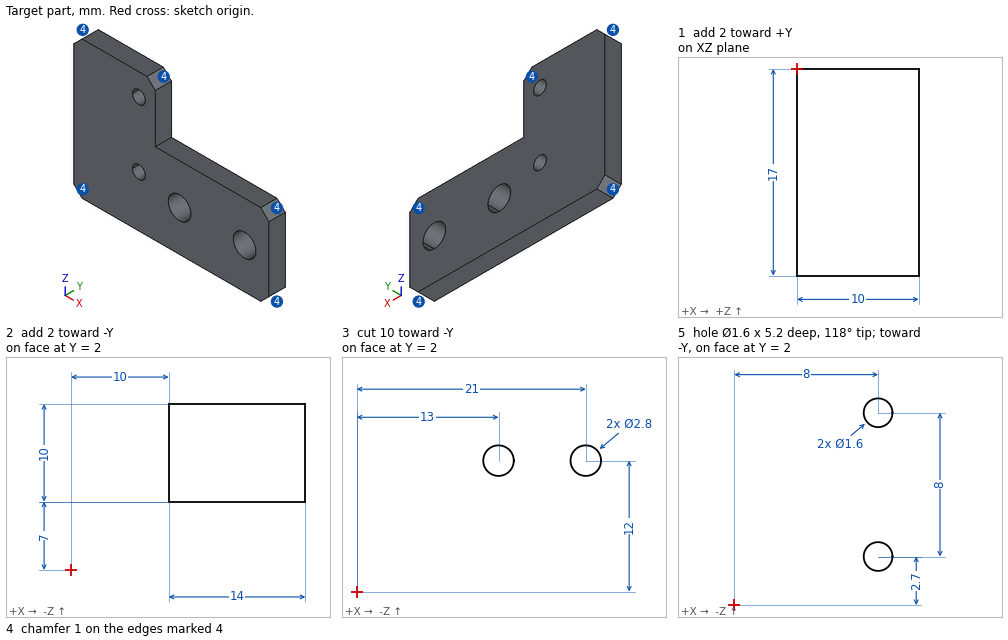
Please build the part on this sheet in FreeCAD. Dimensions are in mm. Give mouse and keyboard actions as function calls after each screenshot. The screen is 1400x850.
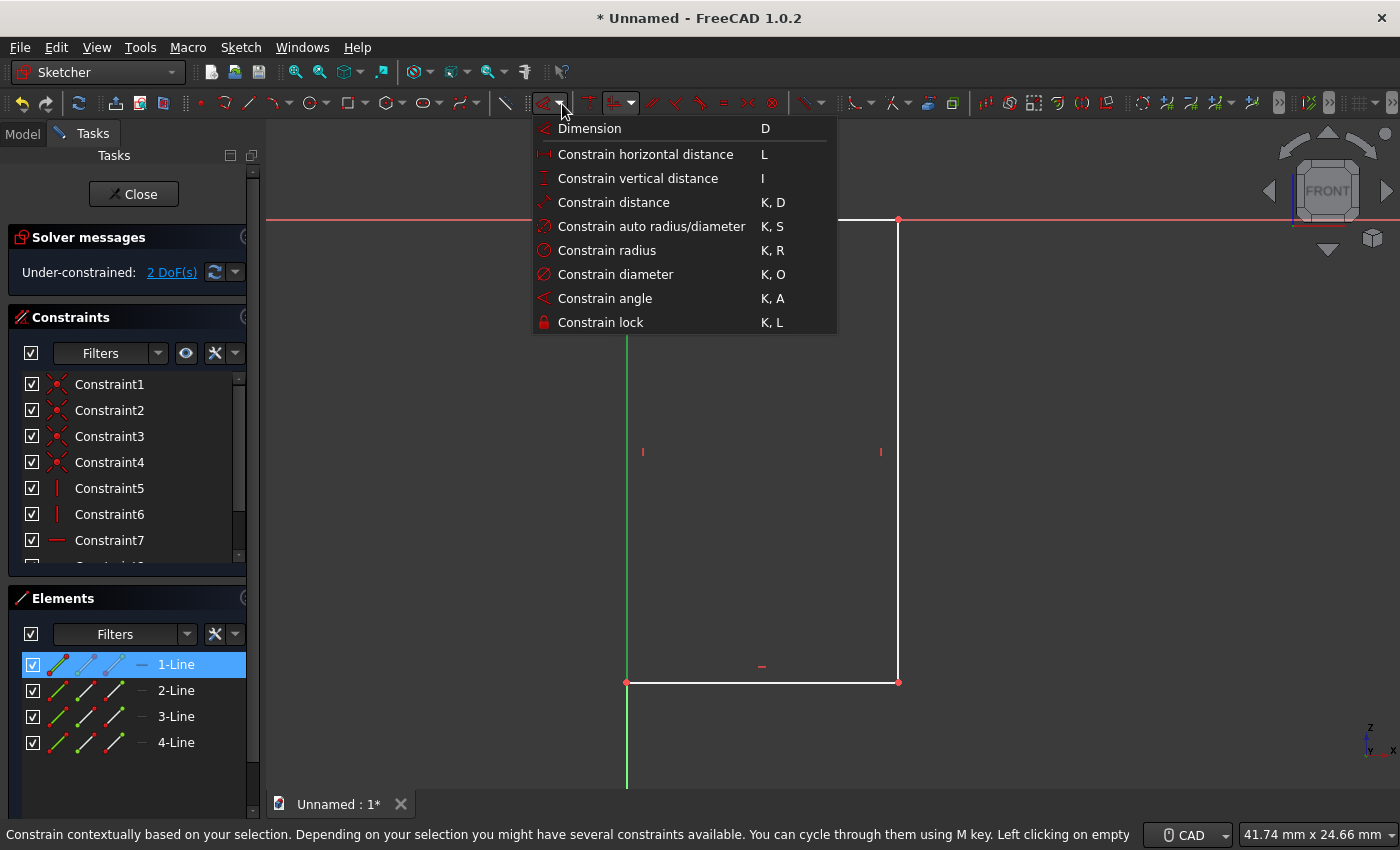
click(685, 178)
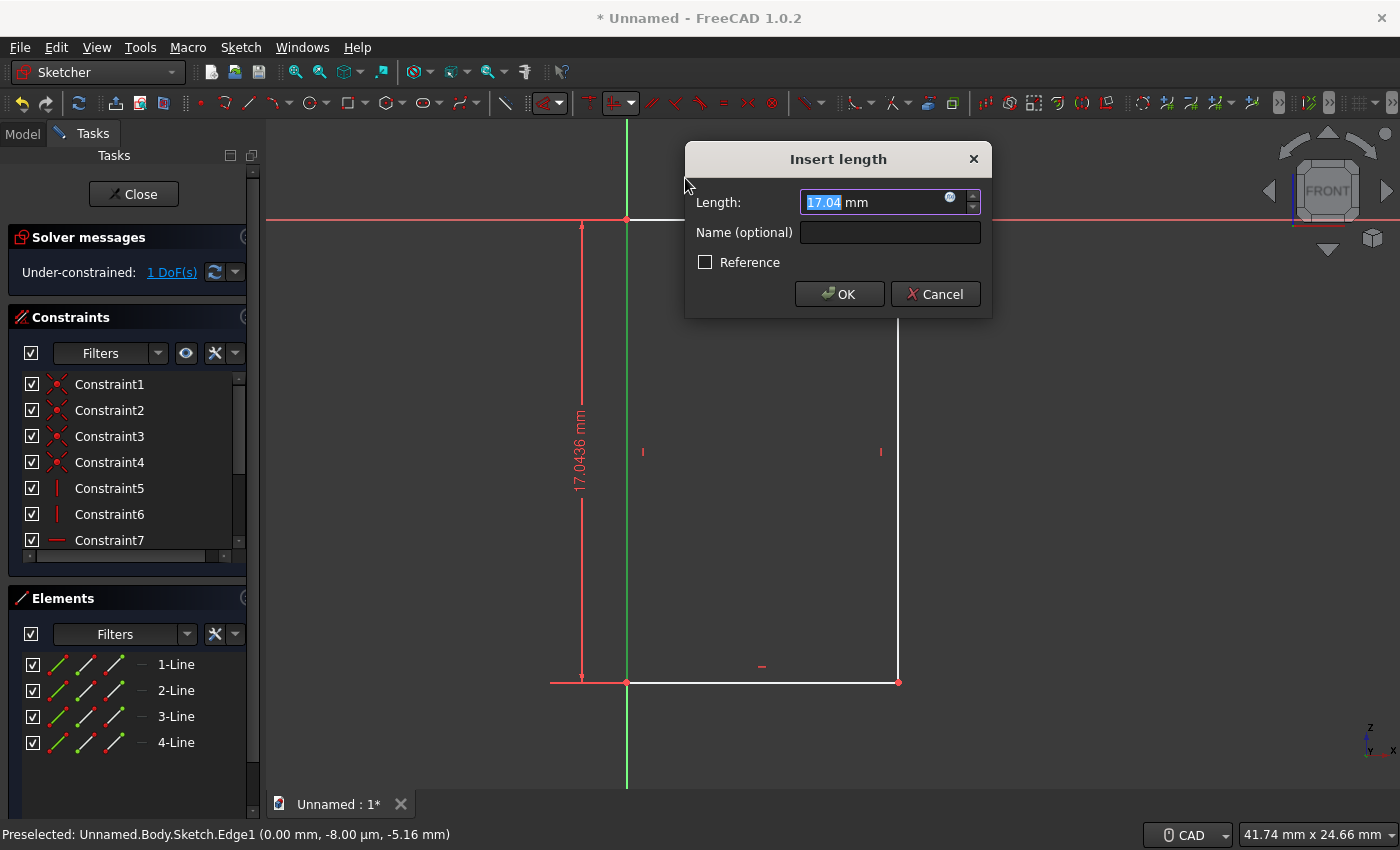
text(17)
key(Return)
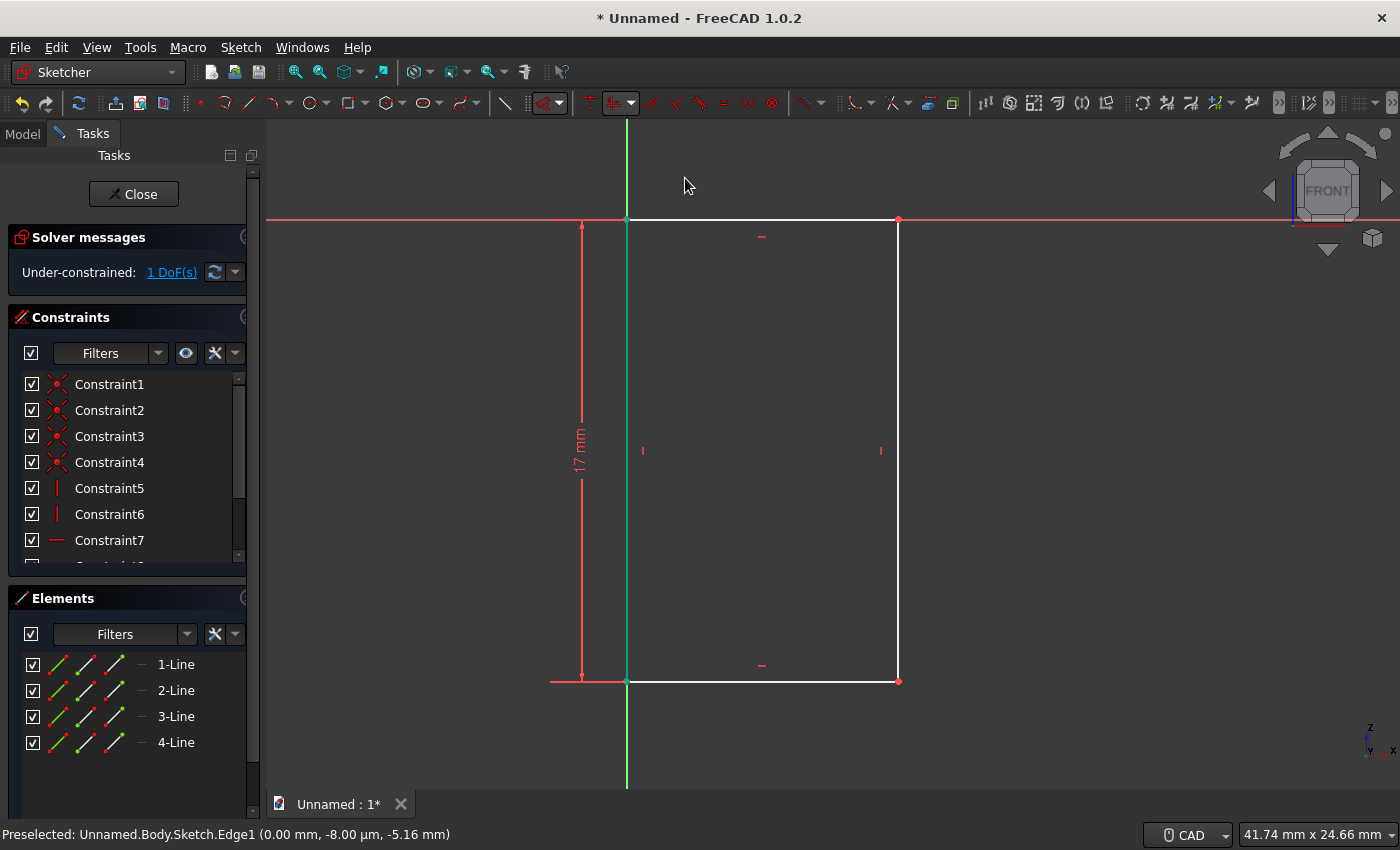
click(708, 682)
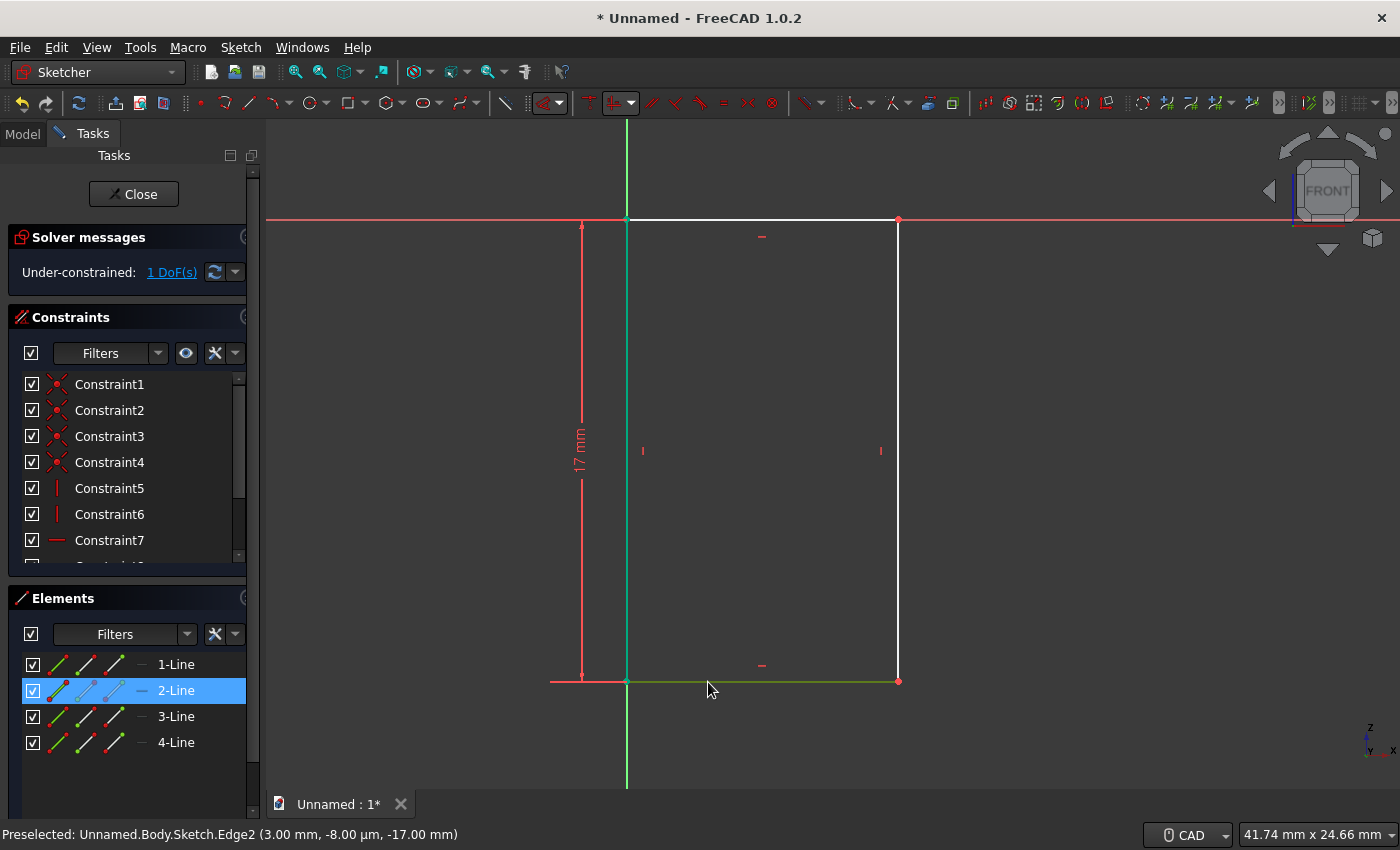
key(l)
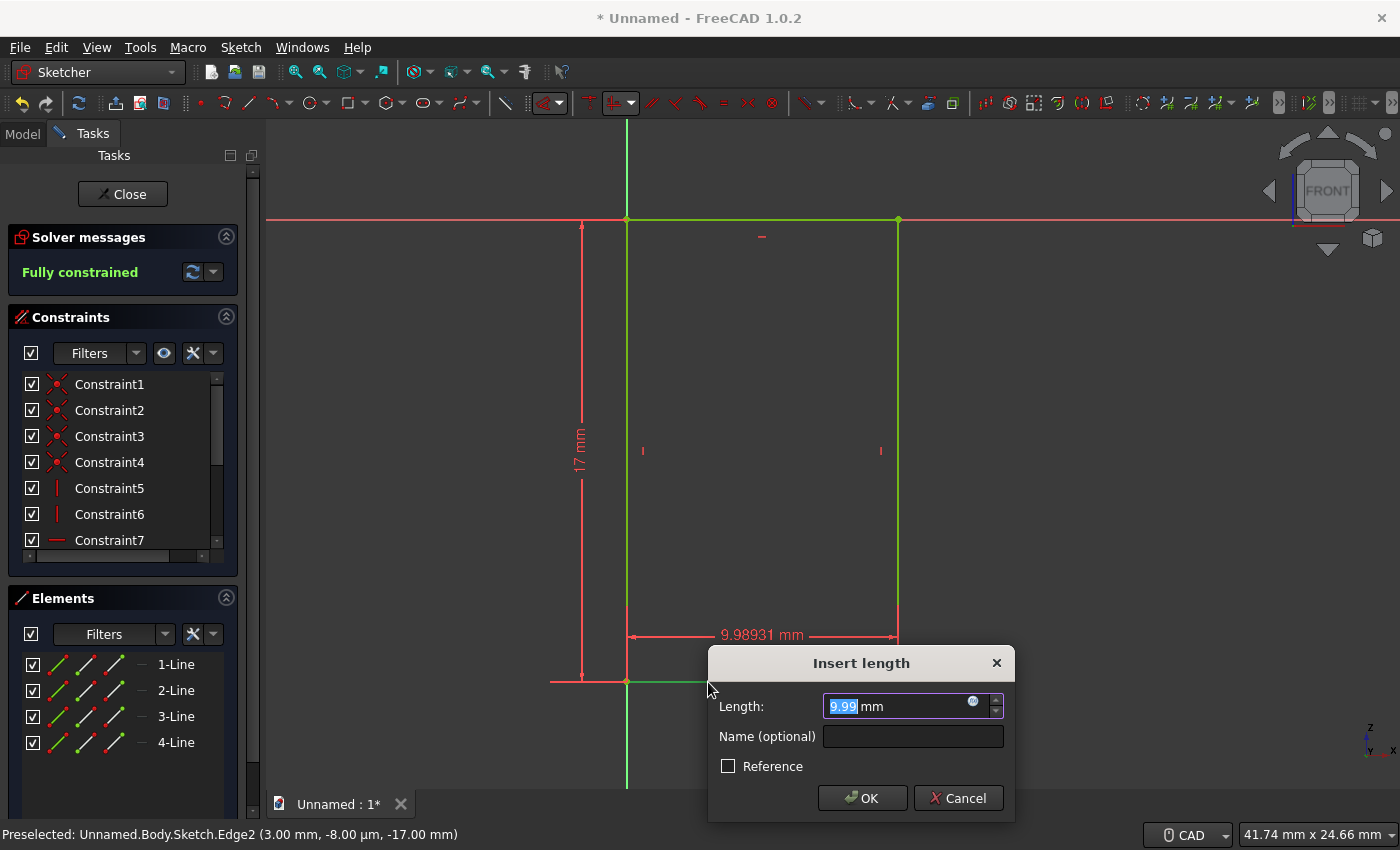
text(10)
key(Return)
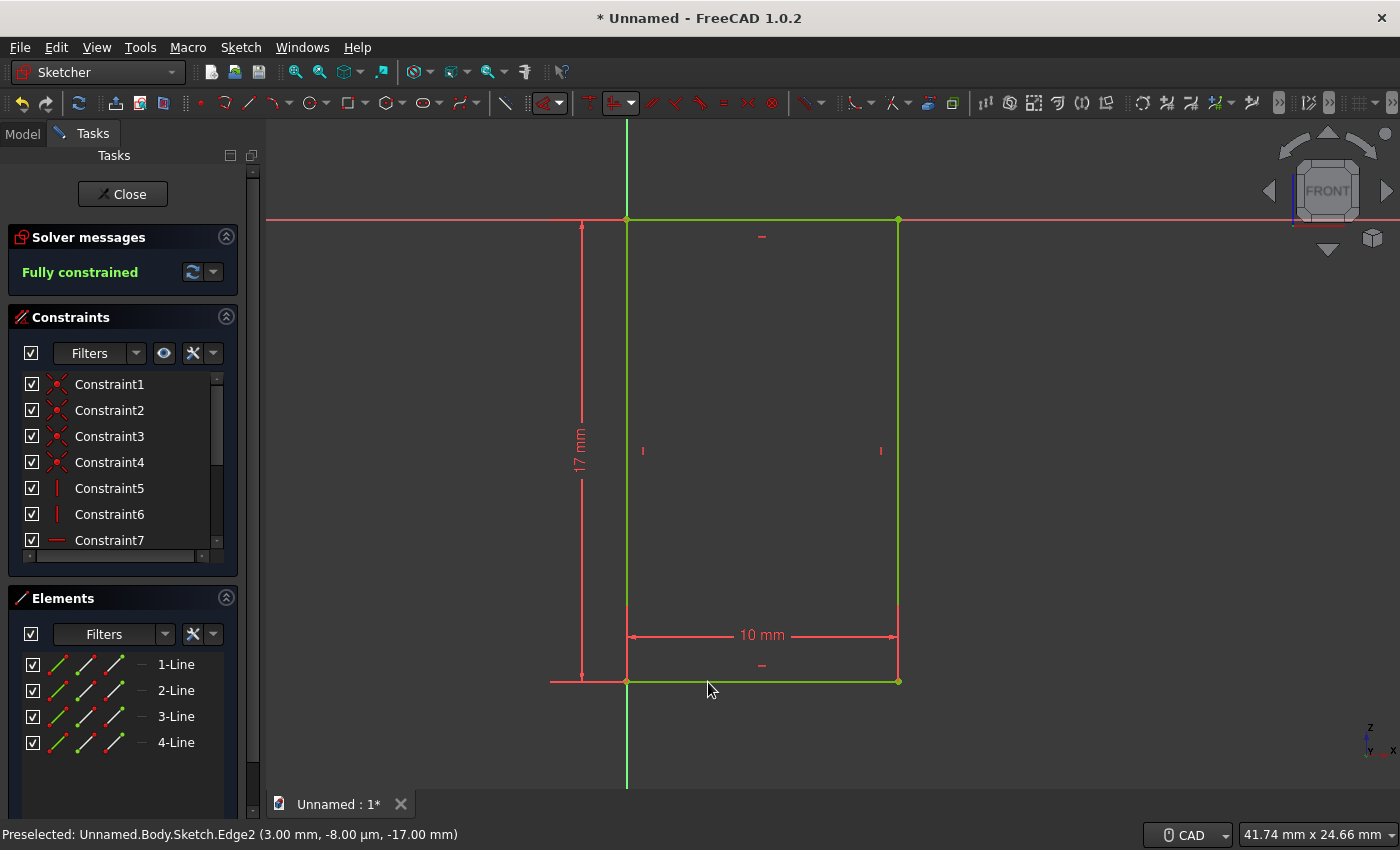
click(123, 194)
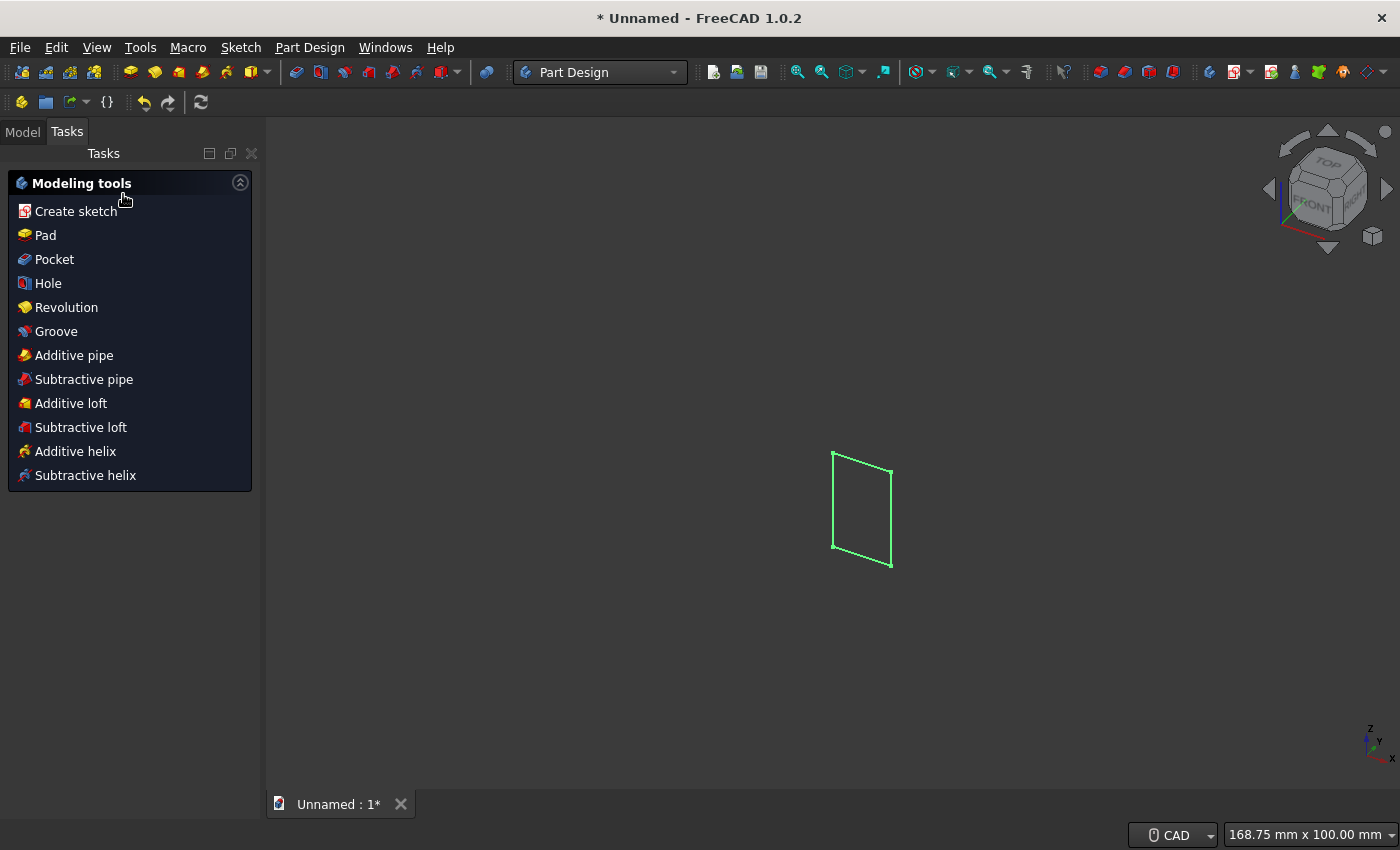
click(132, 72)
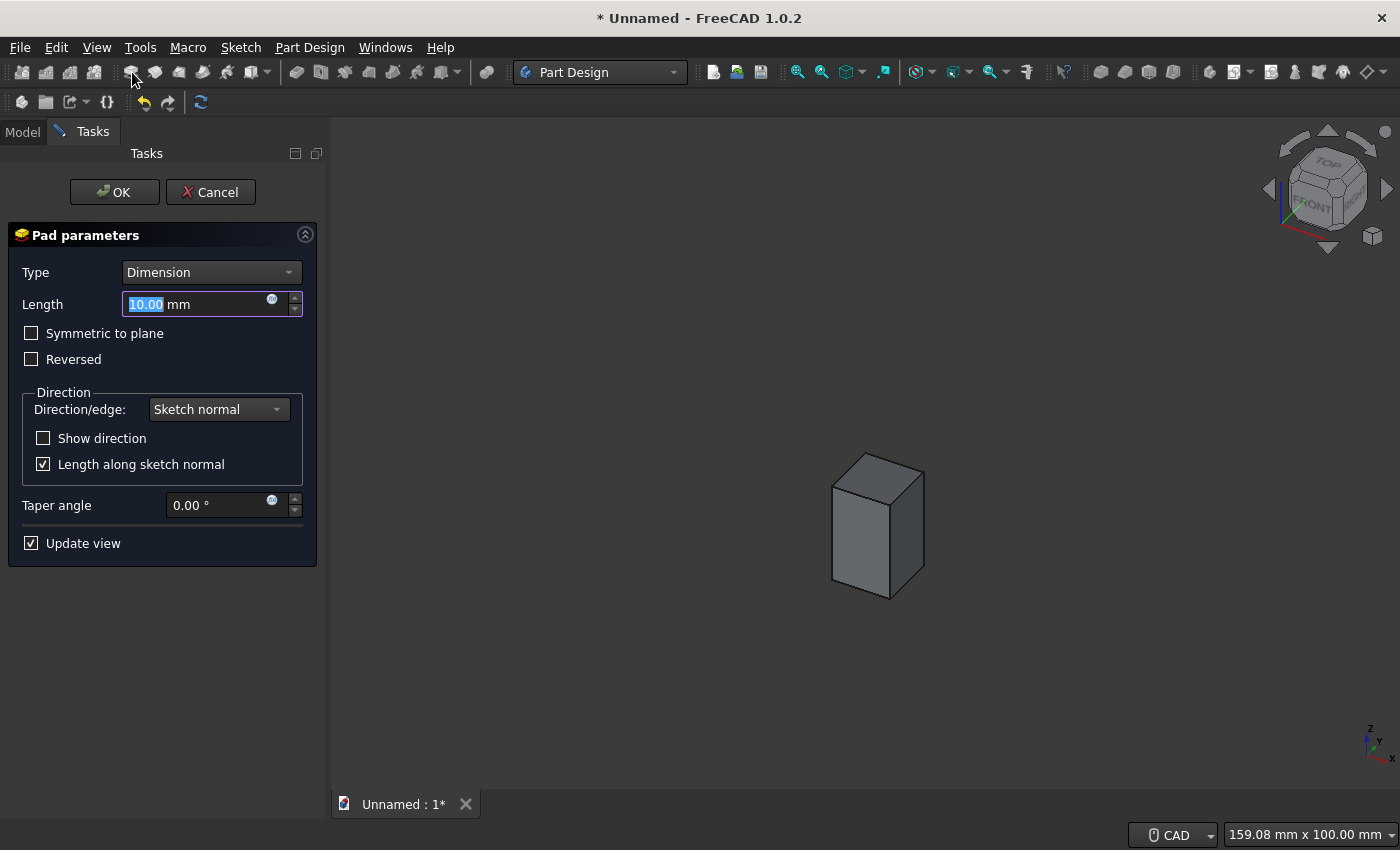
text(2)
key(Tab)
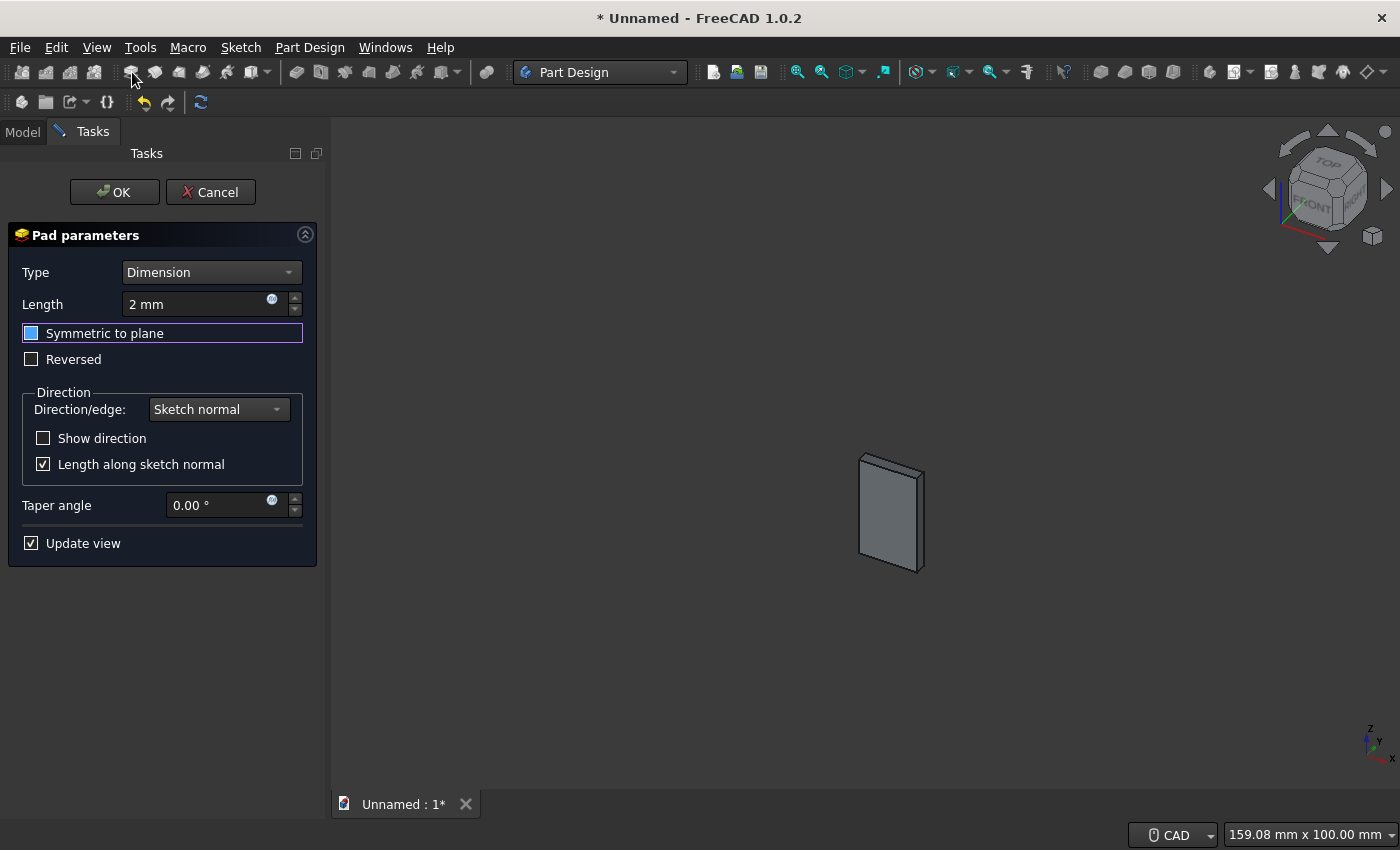
click(30, 359)